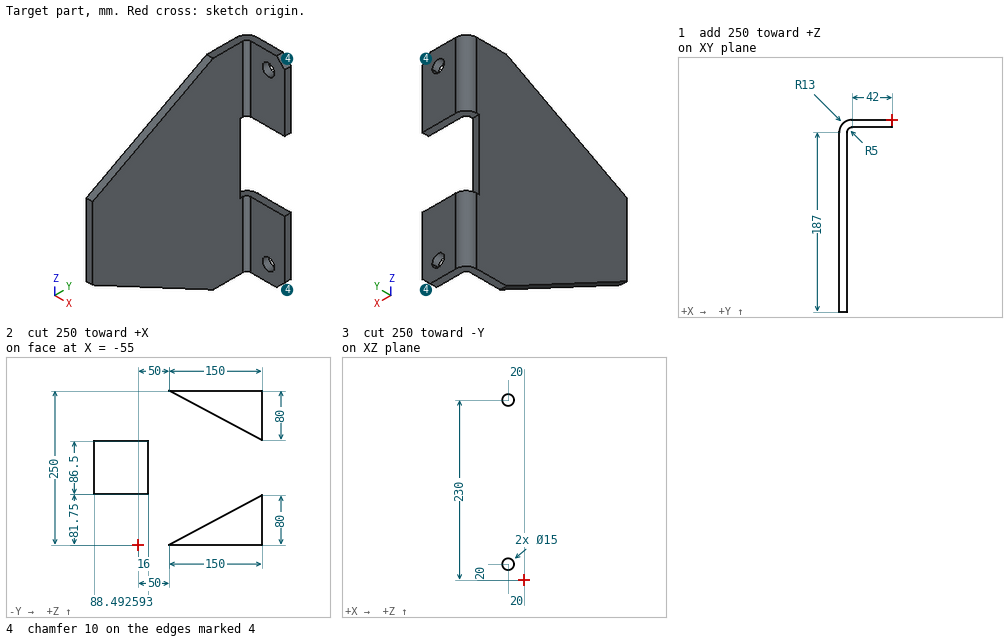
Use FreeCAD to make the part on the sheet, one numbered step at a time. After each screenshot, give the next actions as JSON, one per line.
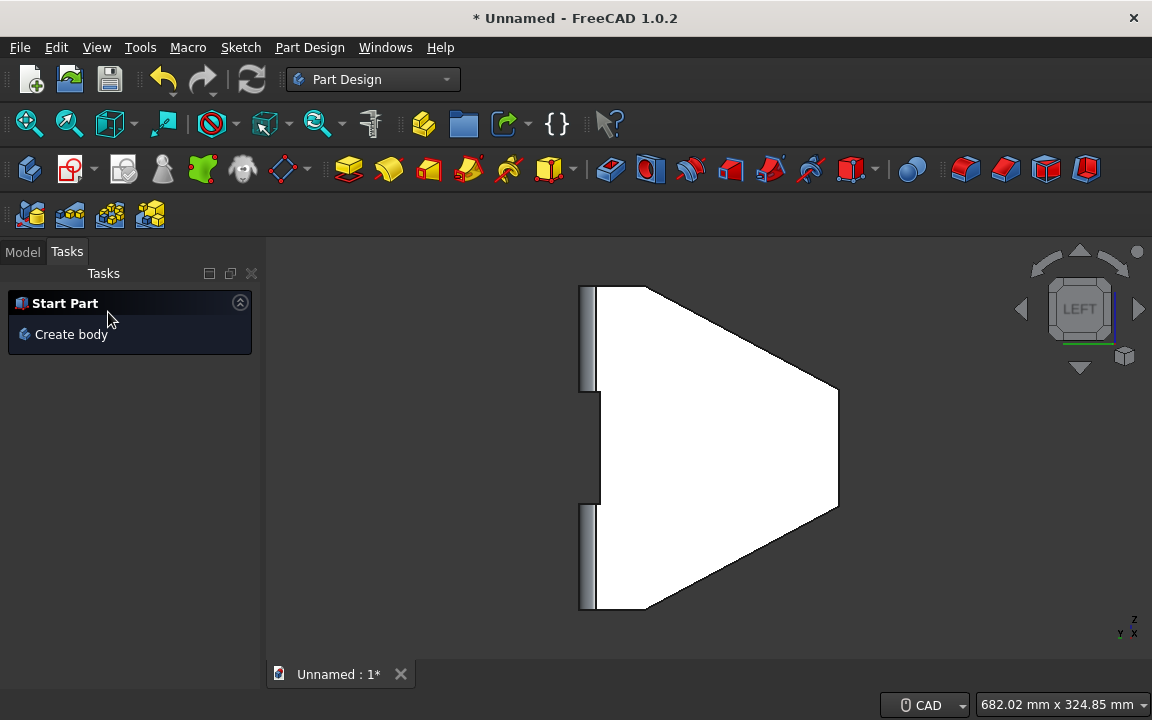
{"action": "left_click", "coordinate": [70, 170]}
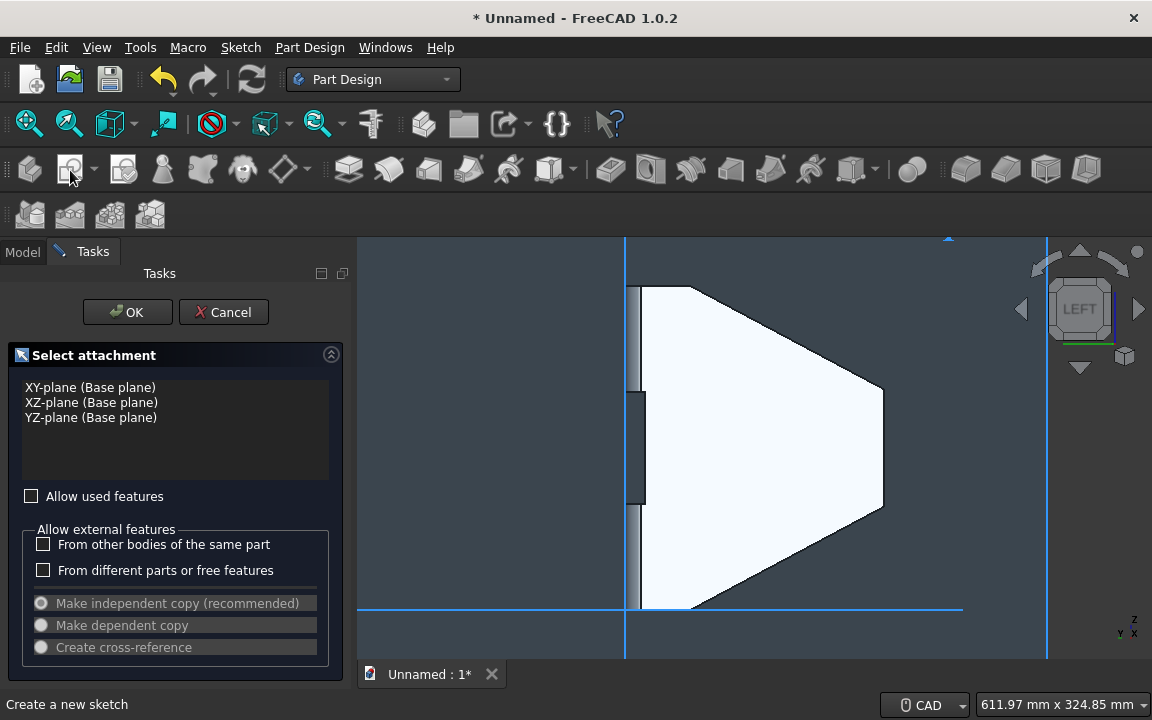
{"action": "left_click", "coordinate": [82, 402]}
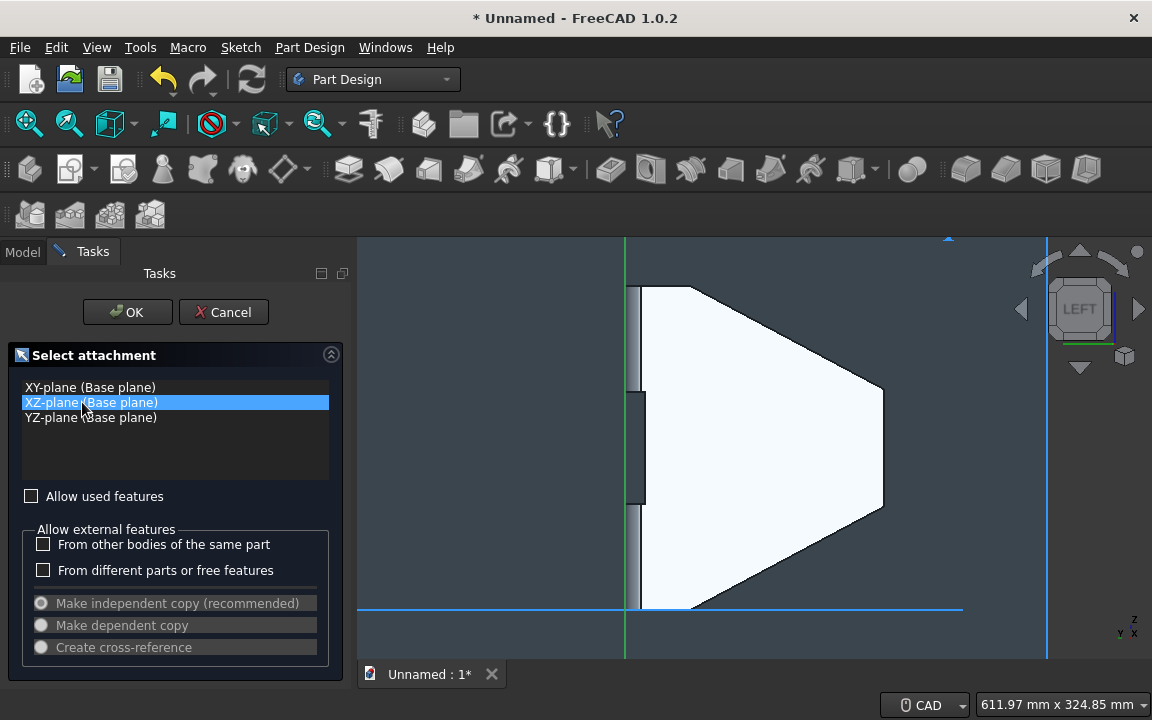
{"action": "left_click", "coordinate": [128, 312]}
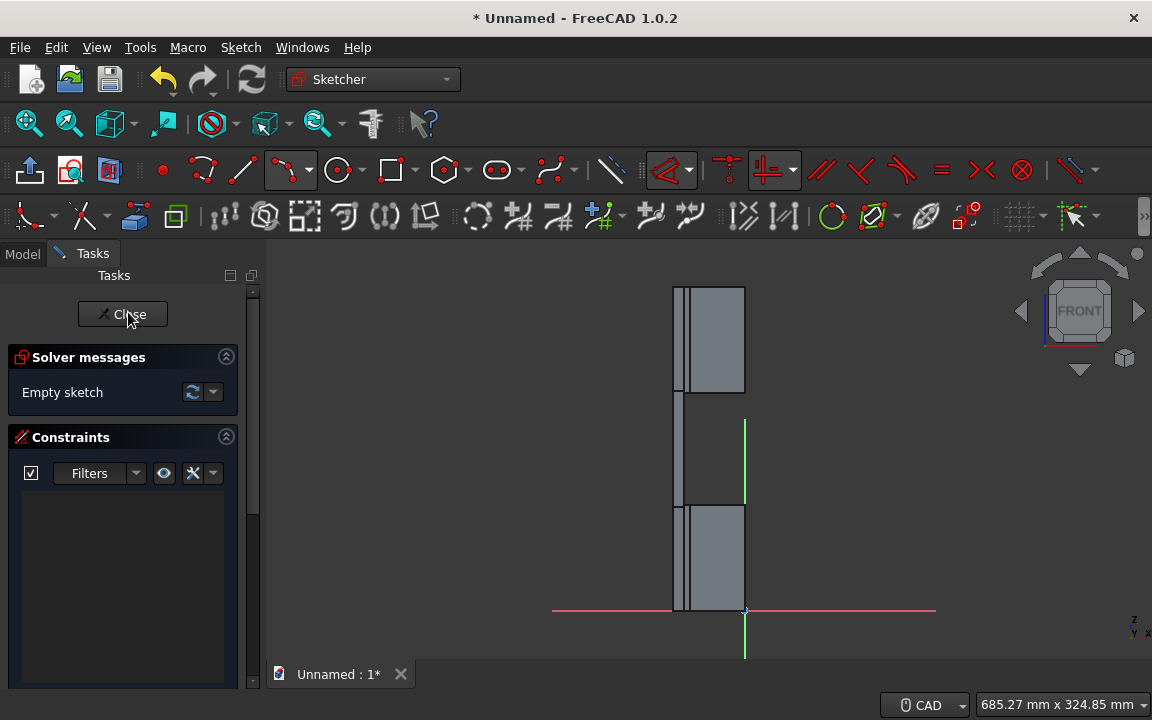
{"action": "left_click", "coordinate": [110, 170]}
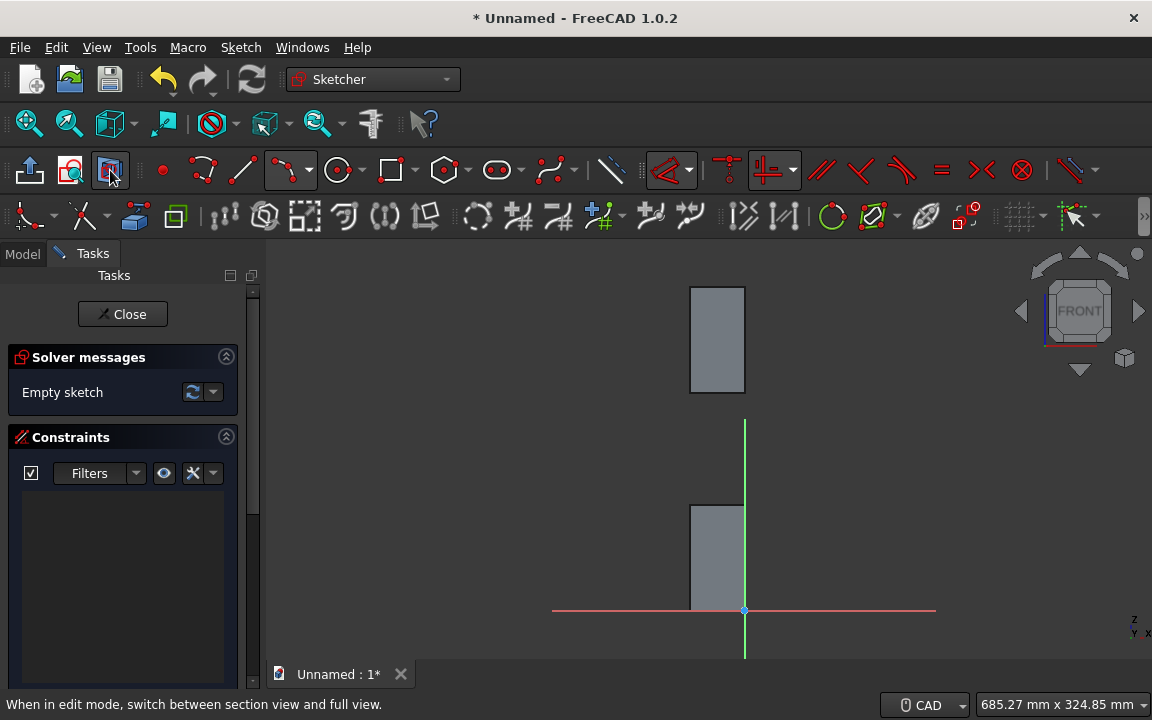
{"action": "scroll", "coordinate": [294, 413], "scroll_direction": "down", "scroll_amount": 1}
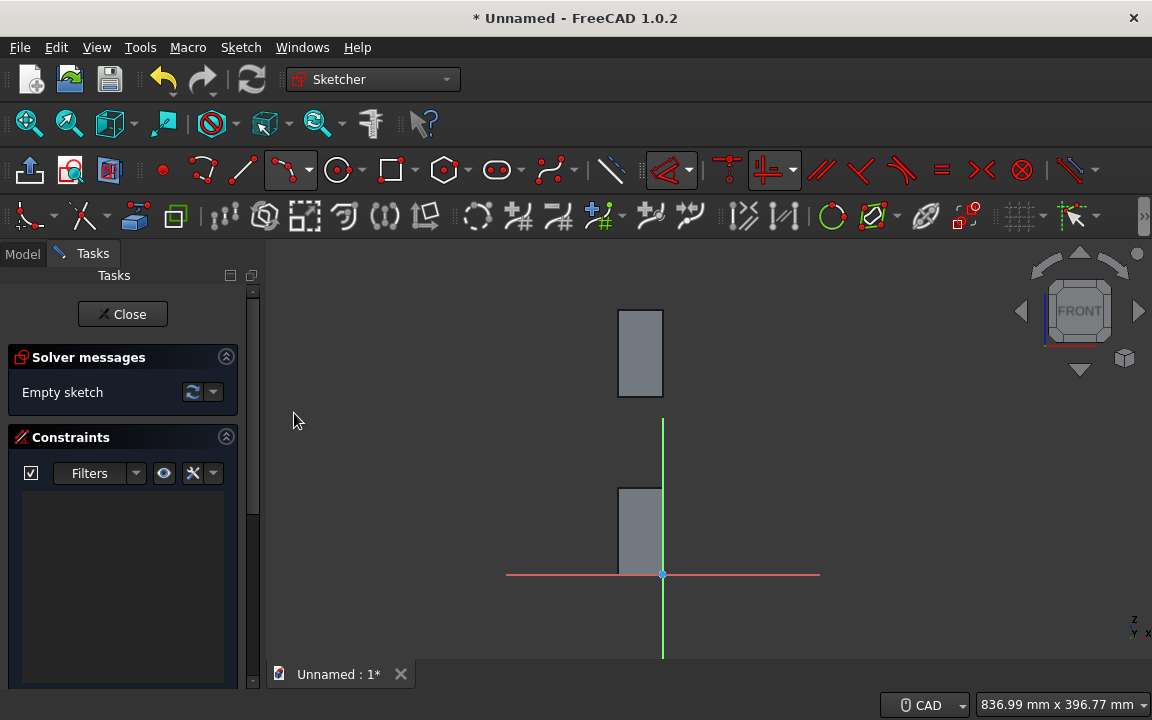
{"action": "left_click", "coordinate": [338, 170]}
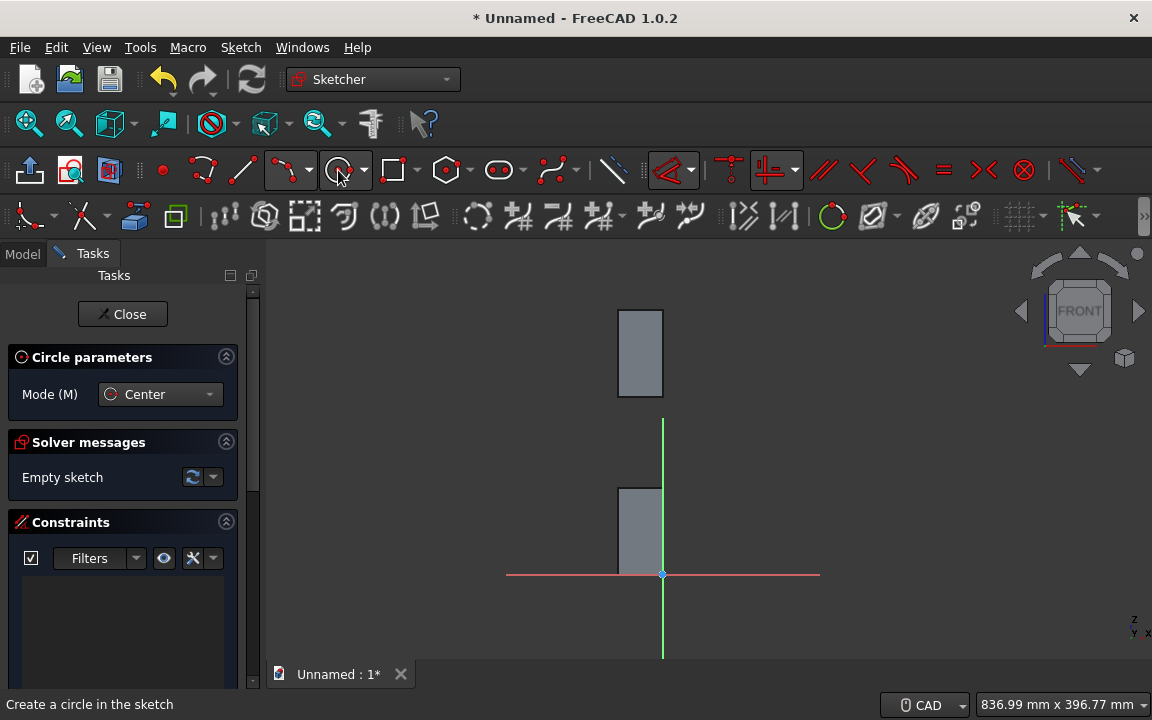
{"action": "scroll", "coordinate": [642, 554], "scroll_direction": "up", "scroll_amount": 6}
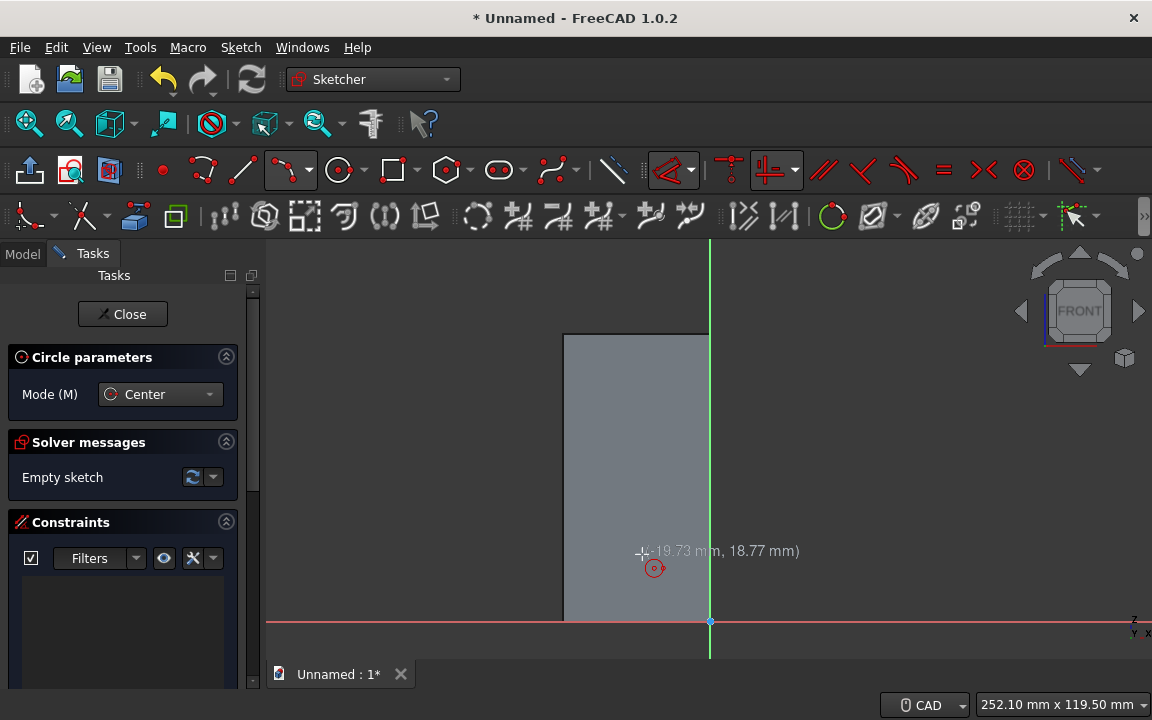
{"action": "left_click", "coordinate": [640, 551]}
{"action": "mouse_move", "coordinate": [659, 533]}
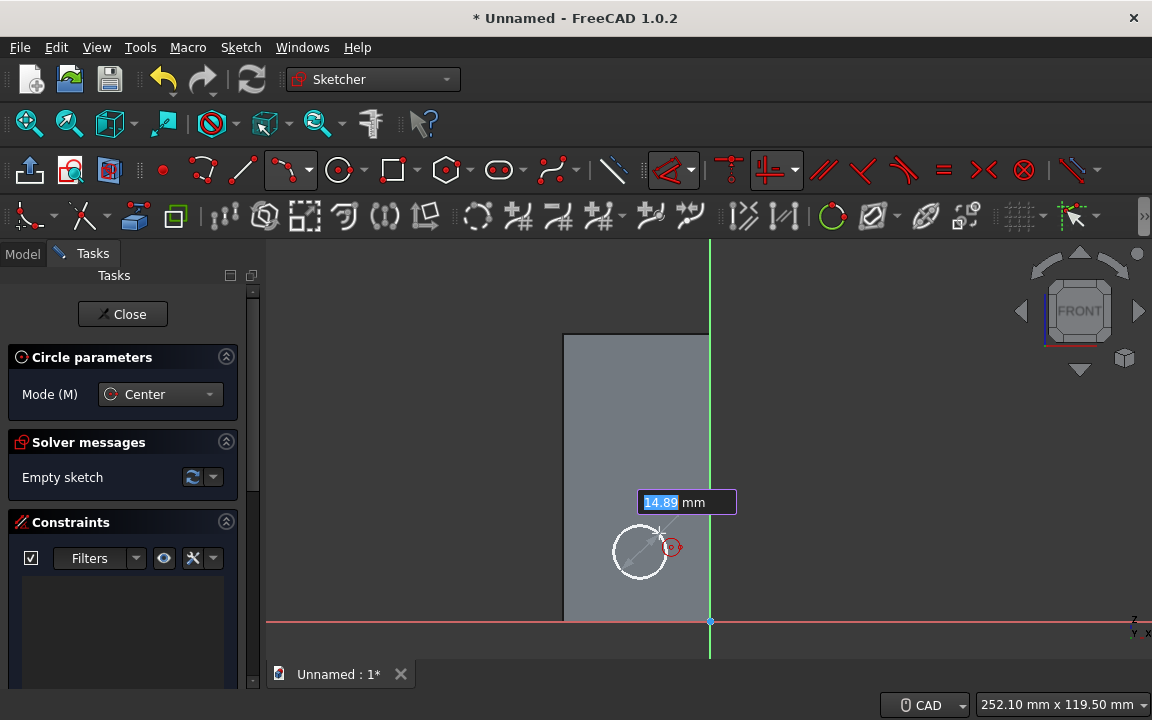
{"action": "type", "text": "15"}
{"action": "key", "text": "Return"}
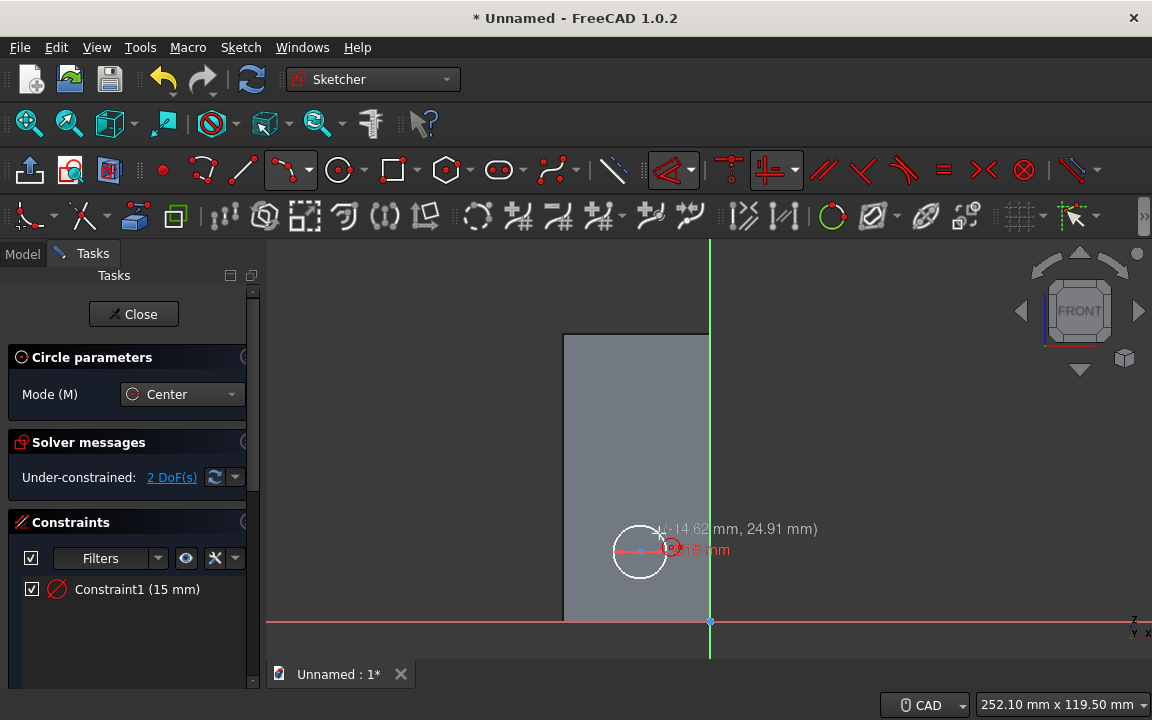
{"action": "scroll", "coordinate": [631, 555], "scroll_direction": "down", "scroll_amount": 6}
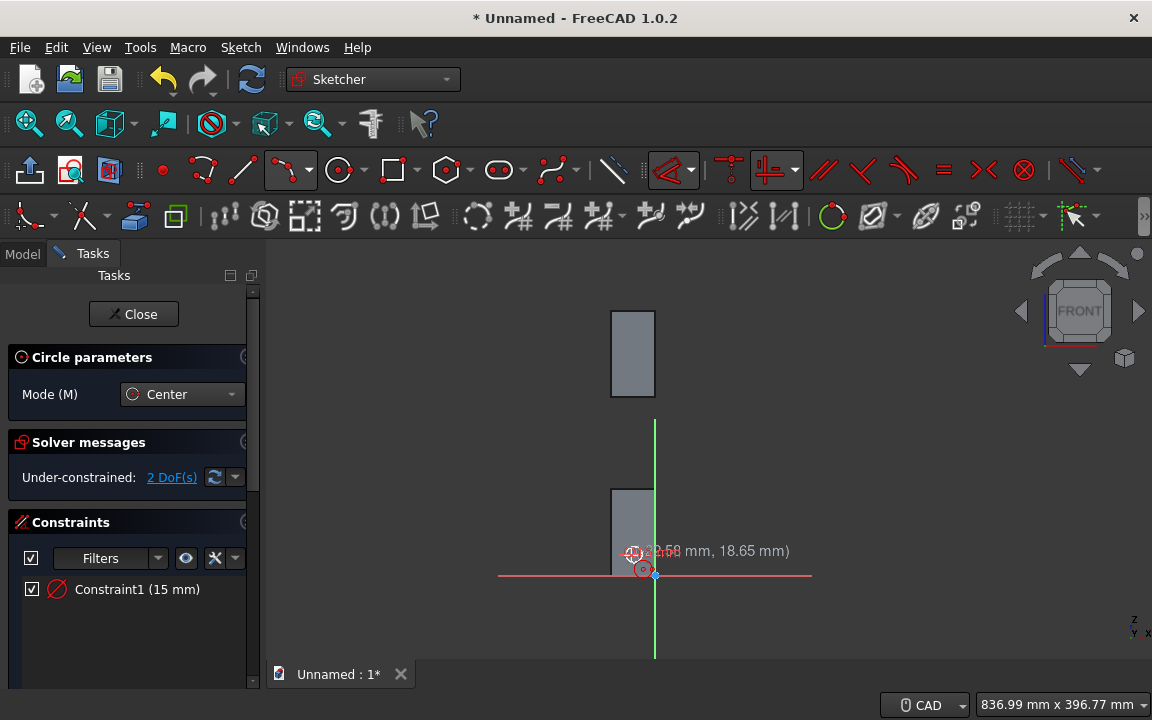
{"action": "scroll", "coordinate": [634, 332], "scroll_direction": "up", "scroll_amount": 6}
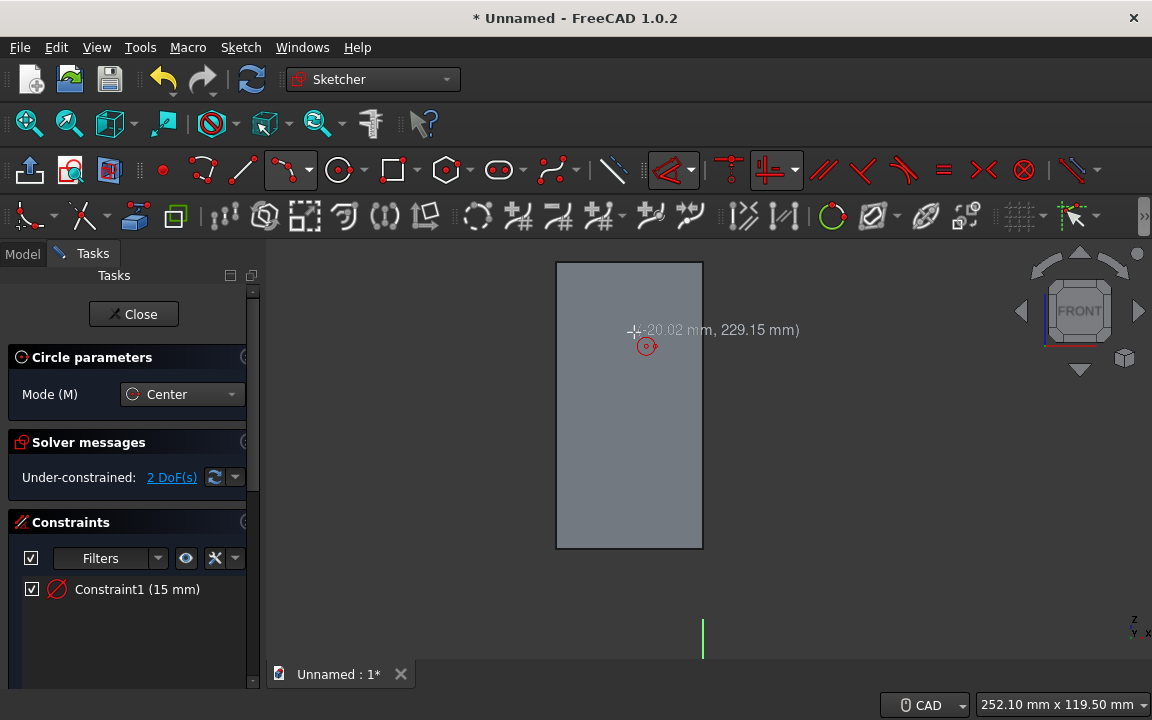
{"action": "left_click", "coordinate": [633, 332]}
{"action": "mouse_move", "coordinate": [652, 313]}